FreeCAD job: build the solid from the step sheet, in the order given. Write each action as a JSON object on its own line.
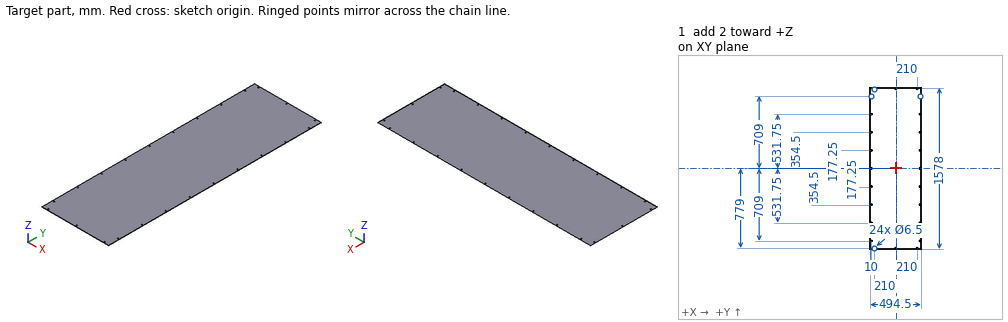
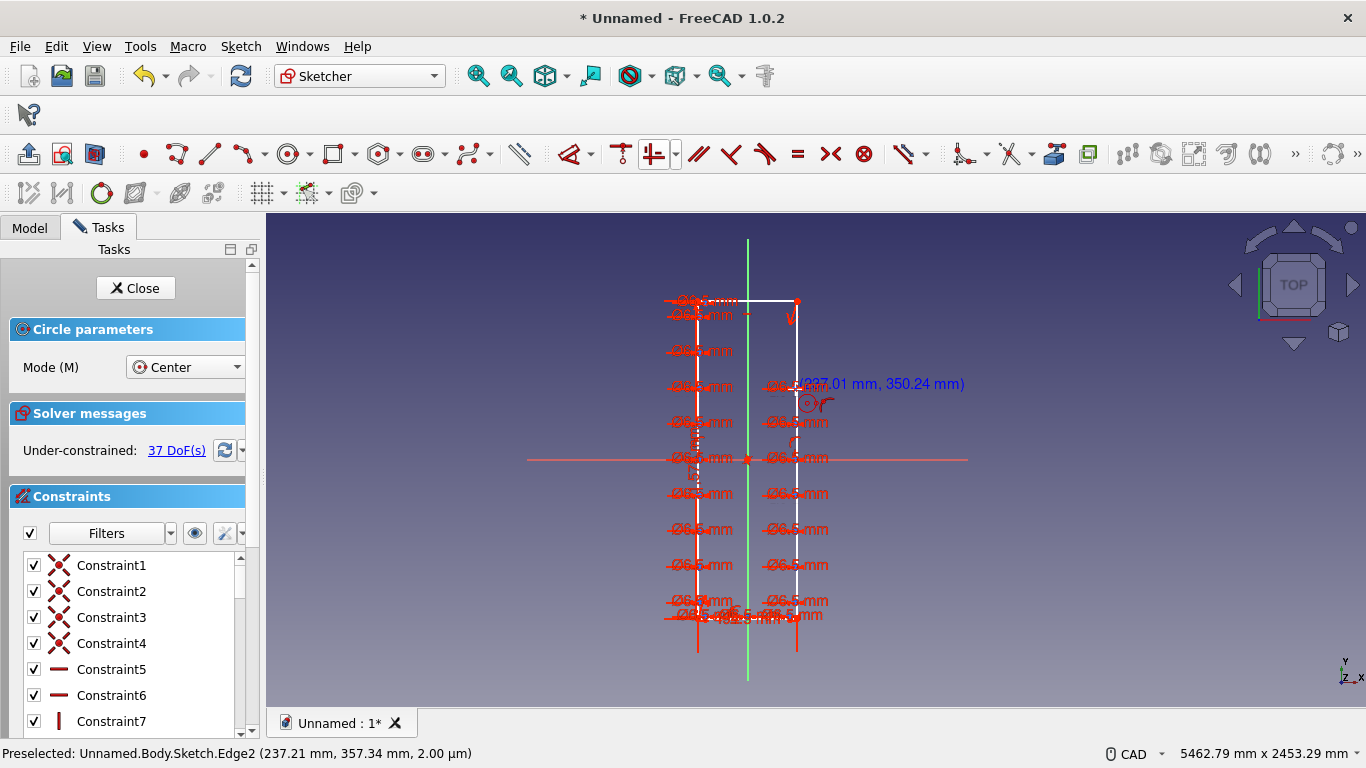
{"action": "scroll", "coordinate": [748, 303], "scroll_direction": "up", "scroll_amount": 18}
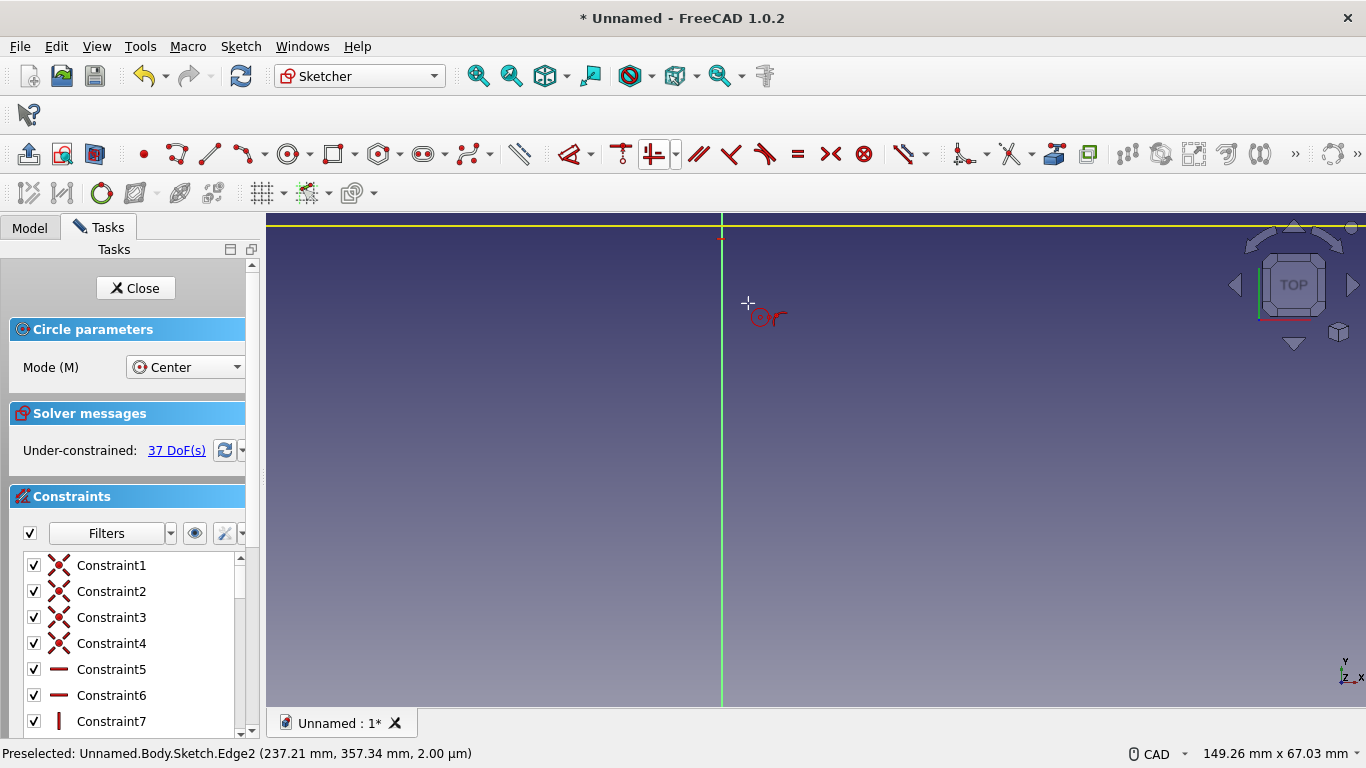
{"action": "scroll", "coordinate": [748, 303], "scroll_direction": "down", "scroll_amount": 18}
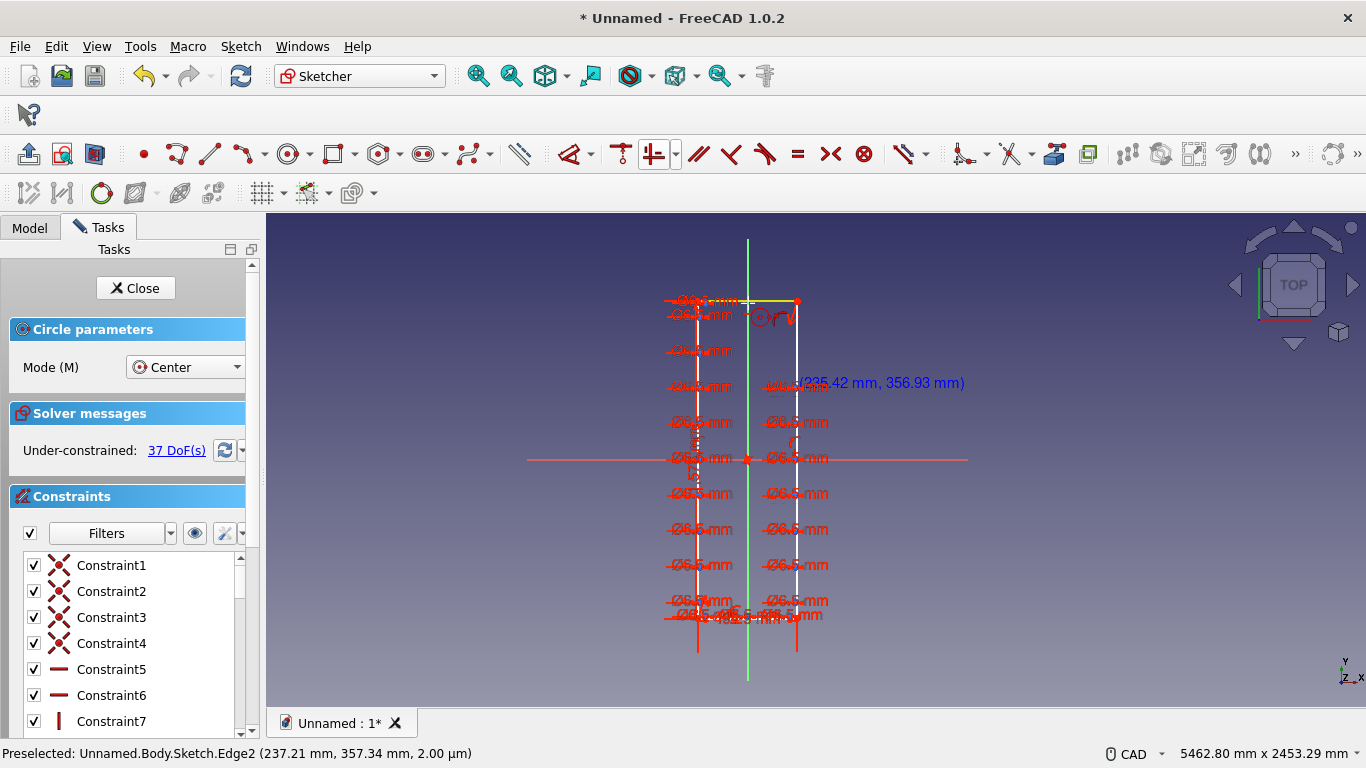
{"action": "scroll", "coordinate": [748, 303], "scroll_direction": "up", "scroll_amount": 11}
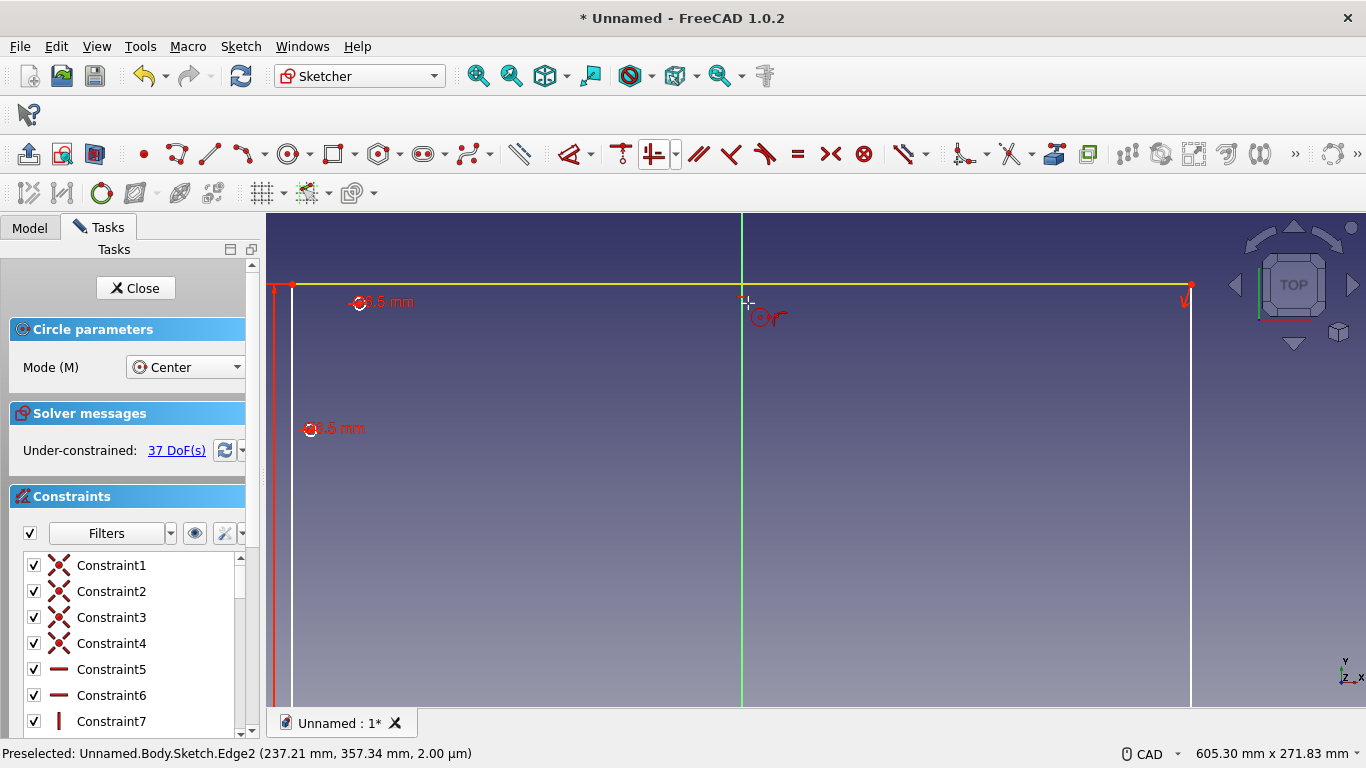
{"action": "left_click", "coordinate": [742, 302]}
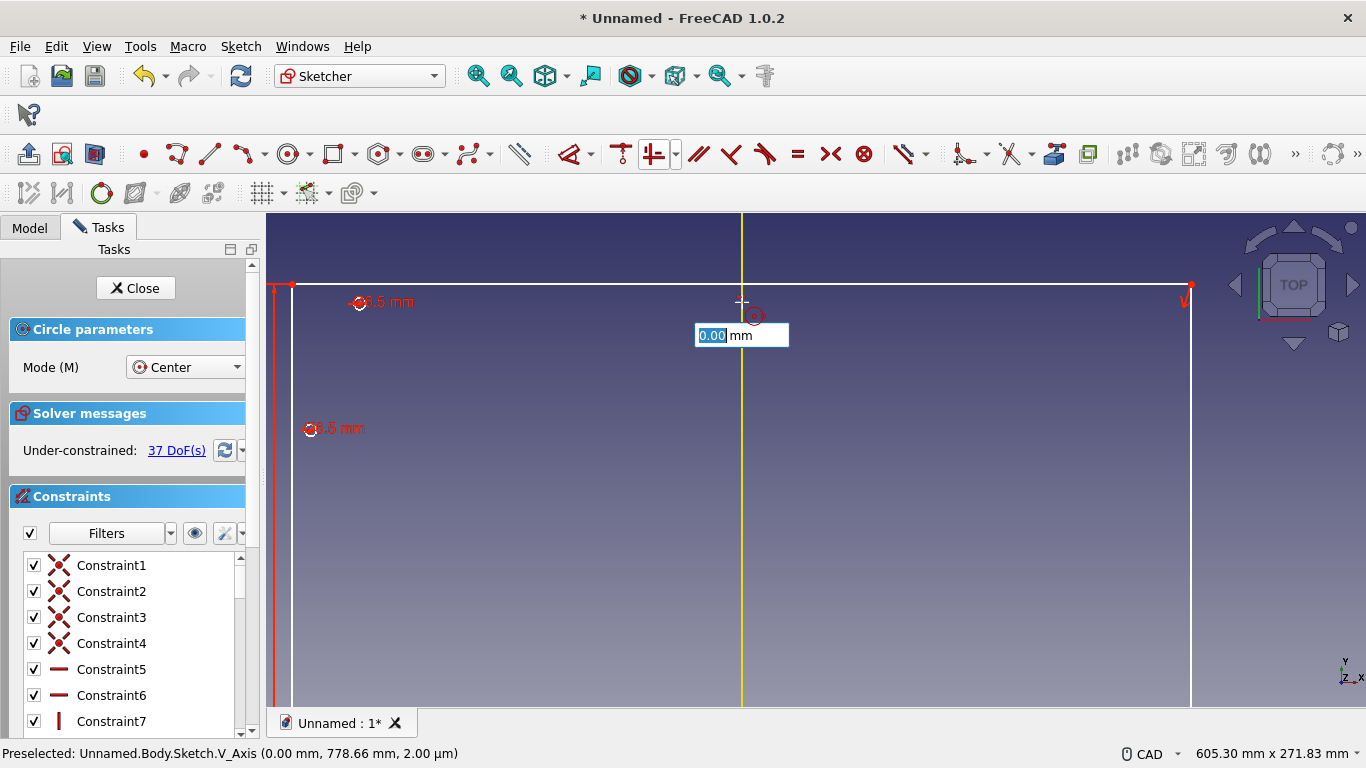
{"action": "scroll", "coordinate": [747, 300], "scroll_direction": "up", "scroll_amount": 6}
{"action": "mouse_move", "coordinate": [747, 301]}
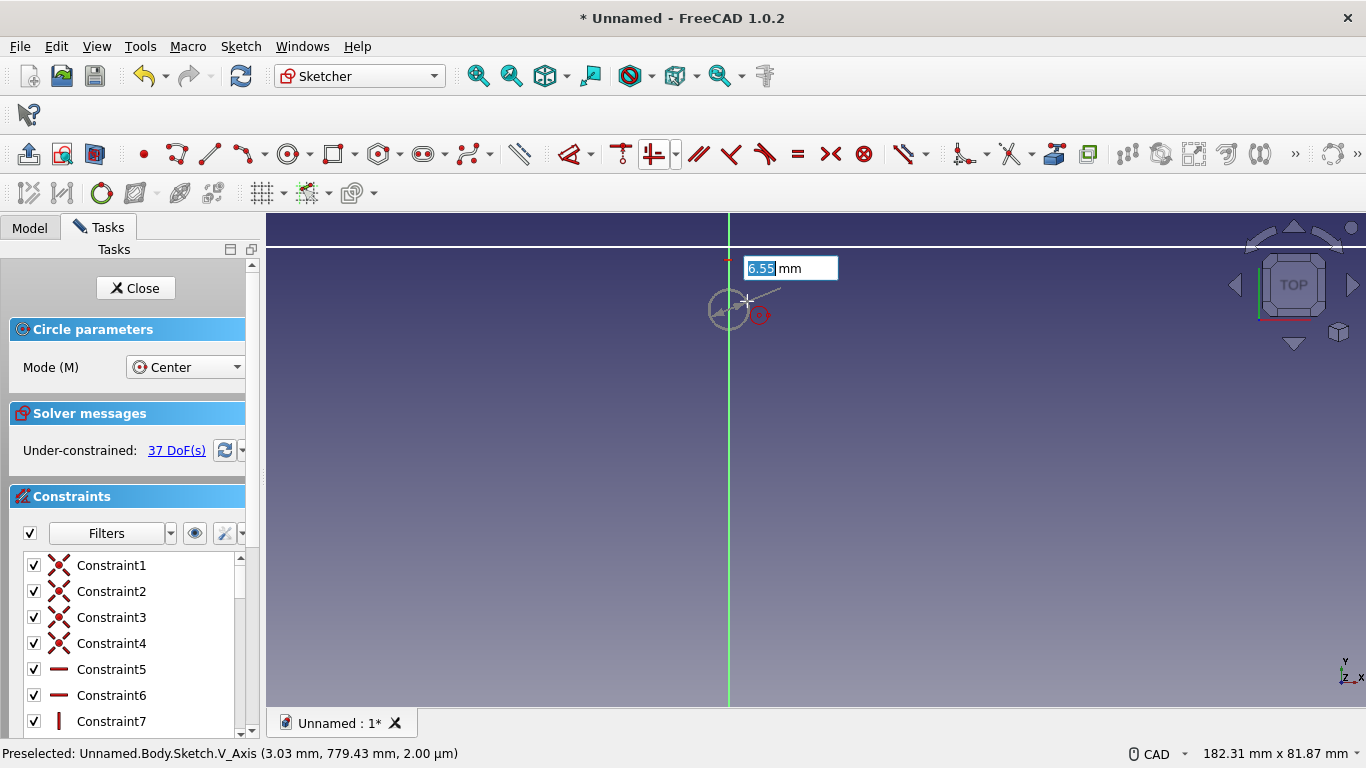
{"action": "type", "text": "6.5"}
{"action": "key", "text": "Return"}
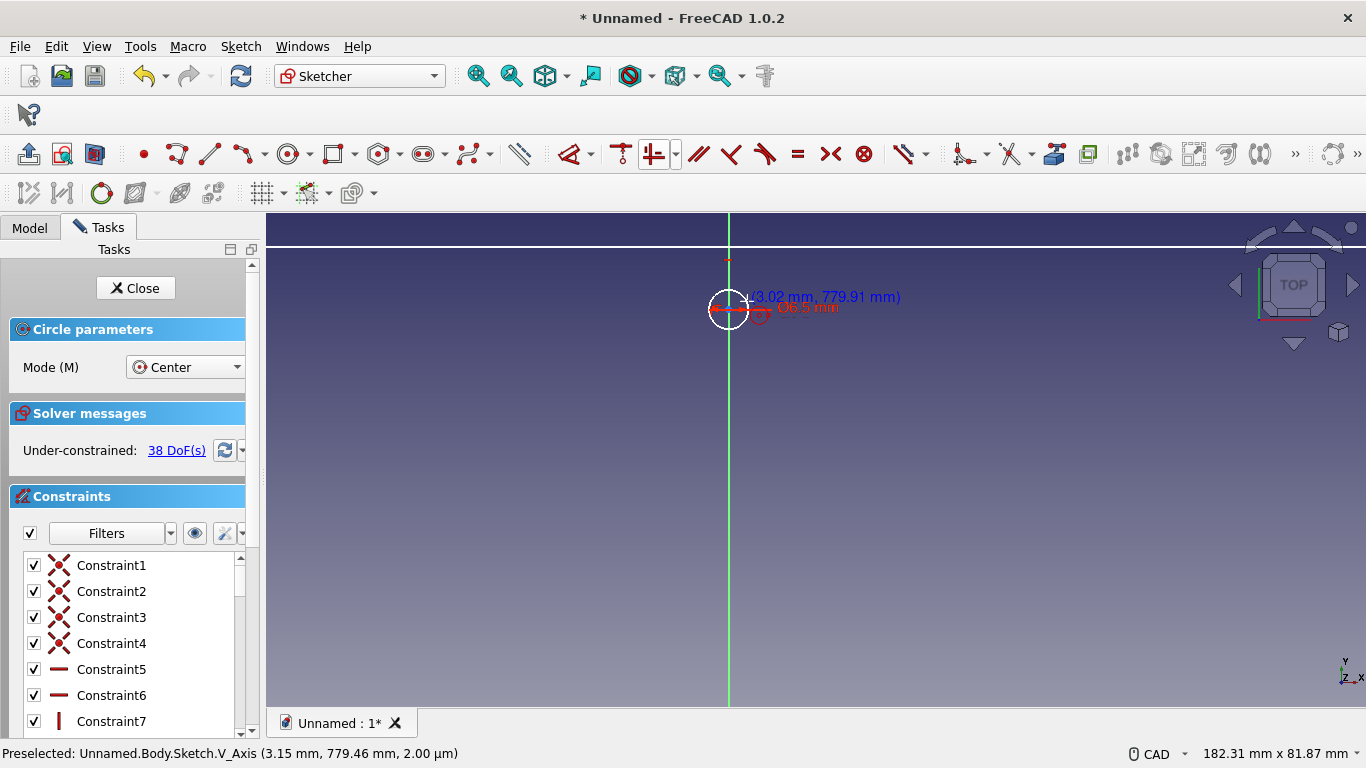
{"action": "scroll", "coordinate": [748, 303], "scroll_direction": "down", "scroll_amount": 17}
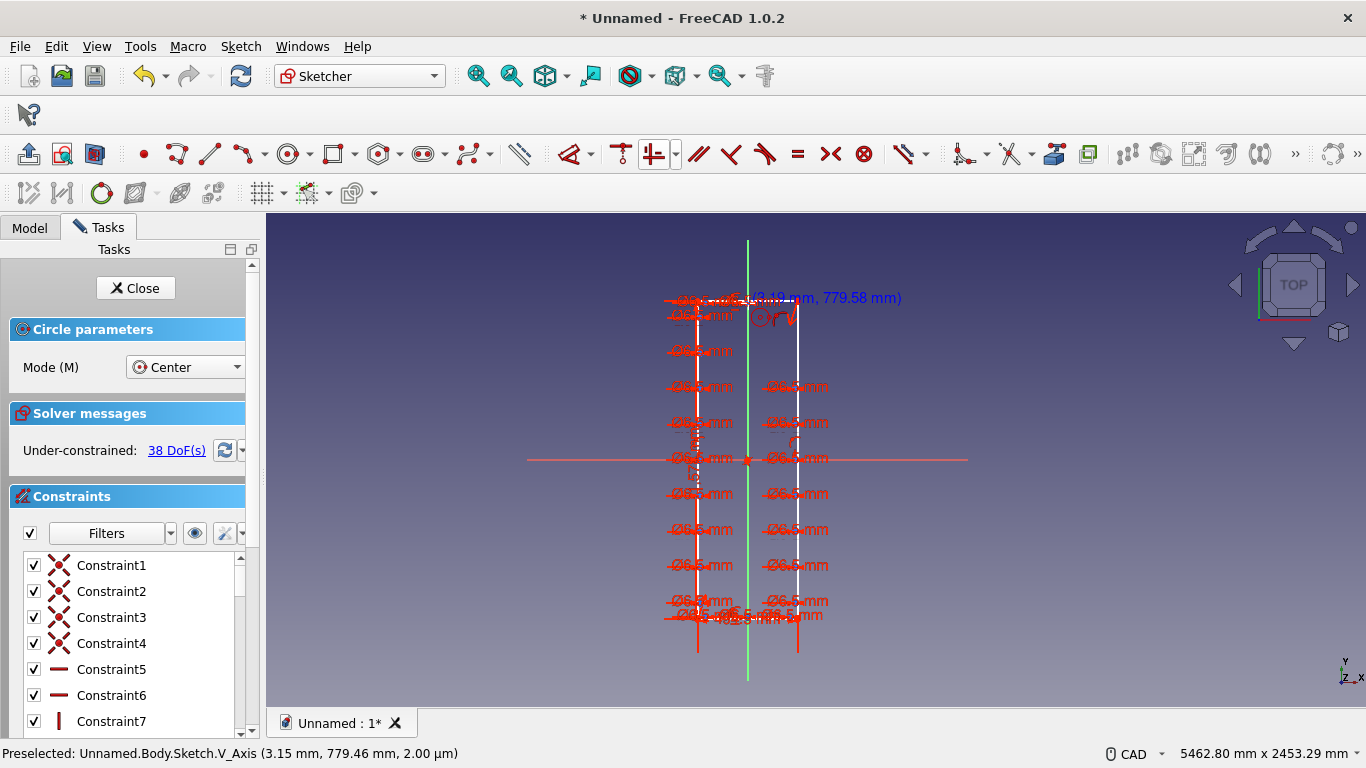
{"action": "scroll", "coordinate": [796, 353], "scroll_direction": "up", "scroll_amount": 18}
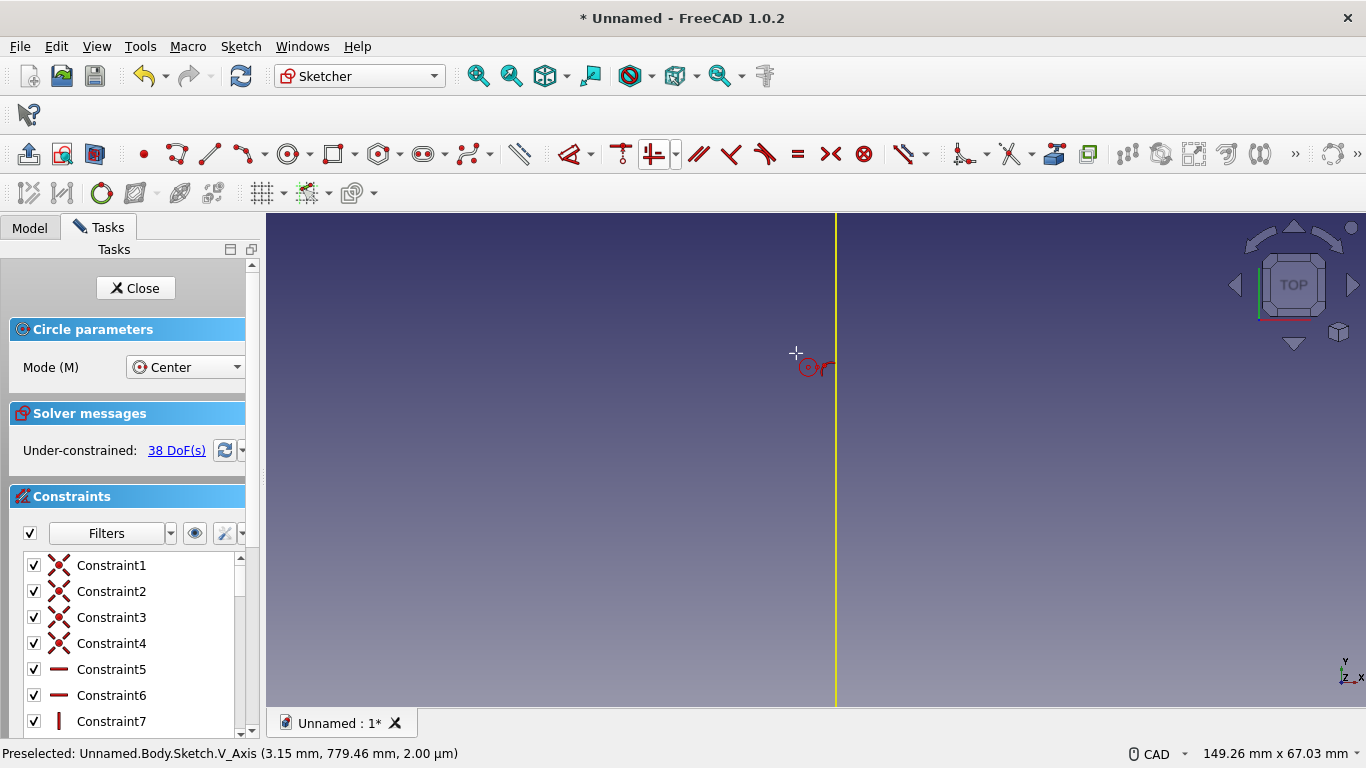
{"action": "scroll", "coordinate": [796, 353], "scroll_direction": "down", "scroll_amount": 18}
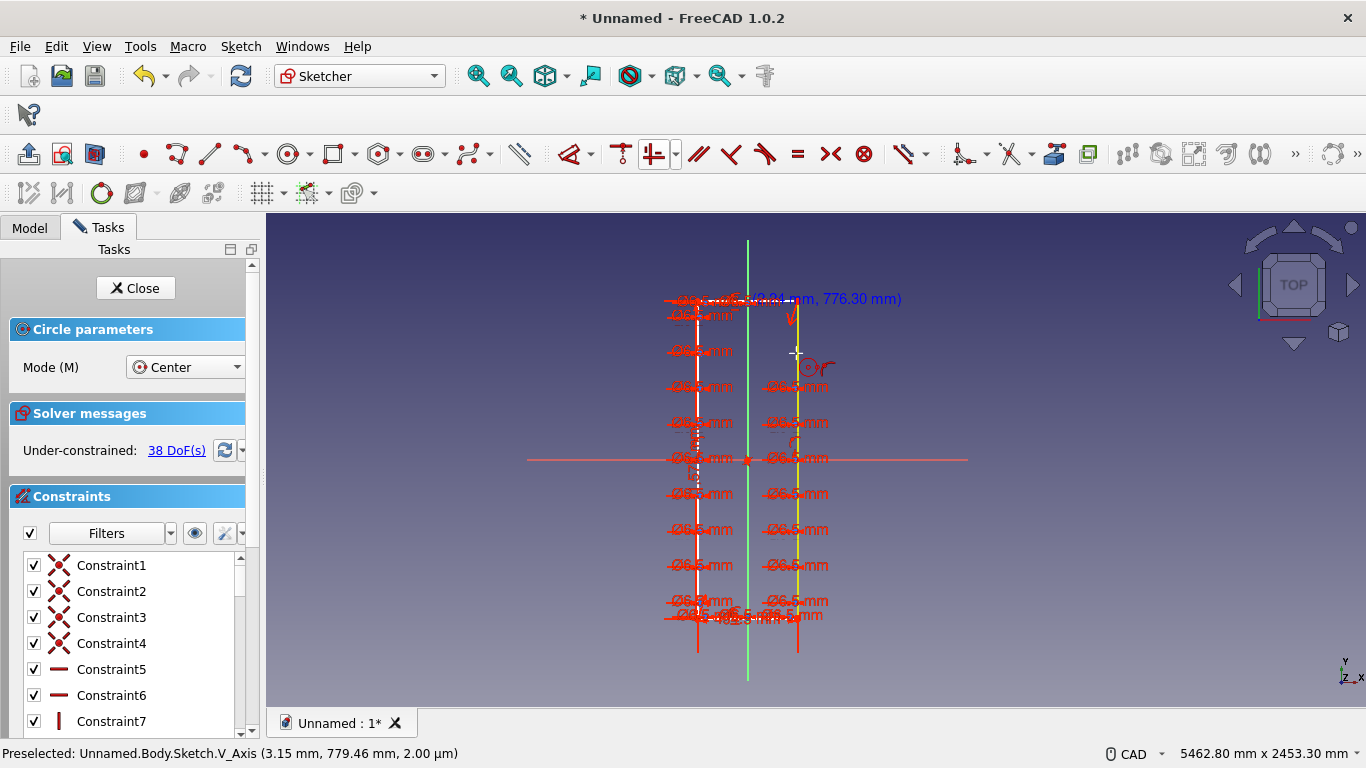
{"action": "scroll", "coordinate": [796, 353], "scroll_direction": "up", "scroll_amount": 11}